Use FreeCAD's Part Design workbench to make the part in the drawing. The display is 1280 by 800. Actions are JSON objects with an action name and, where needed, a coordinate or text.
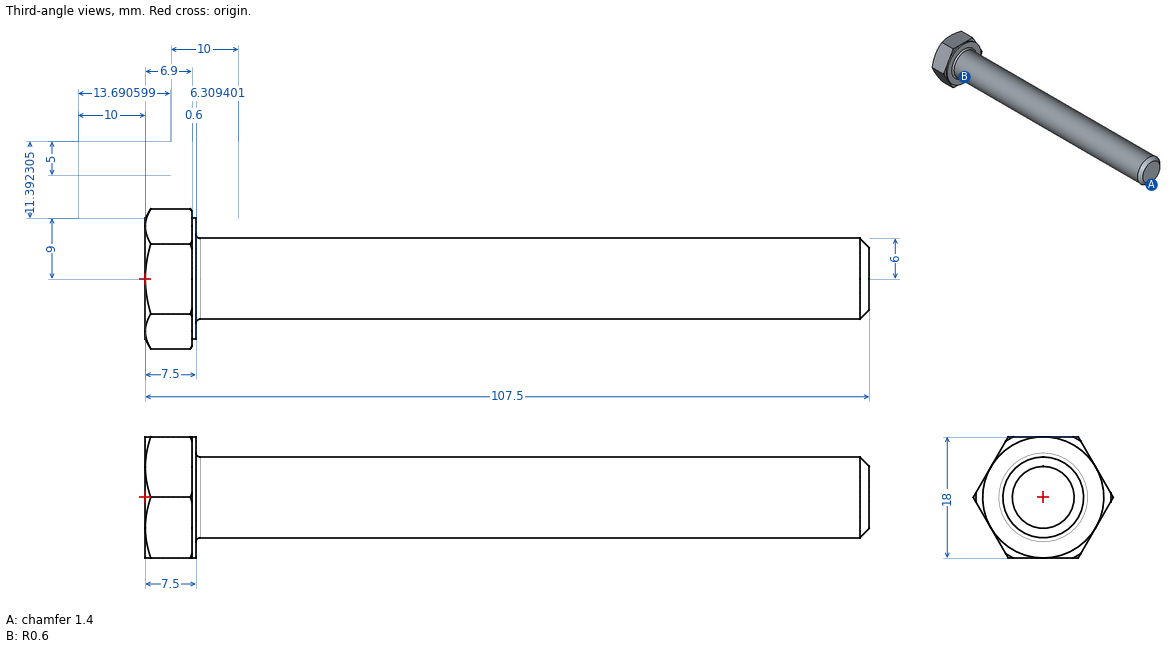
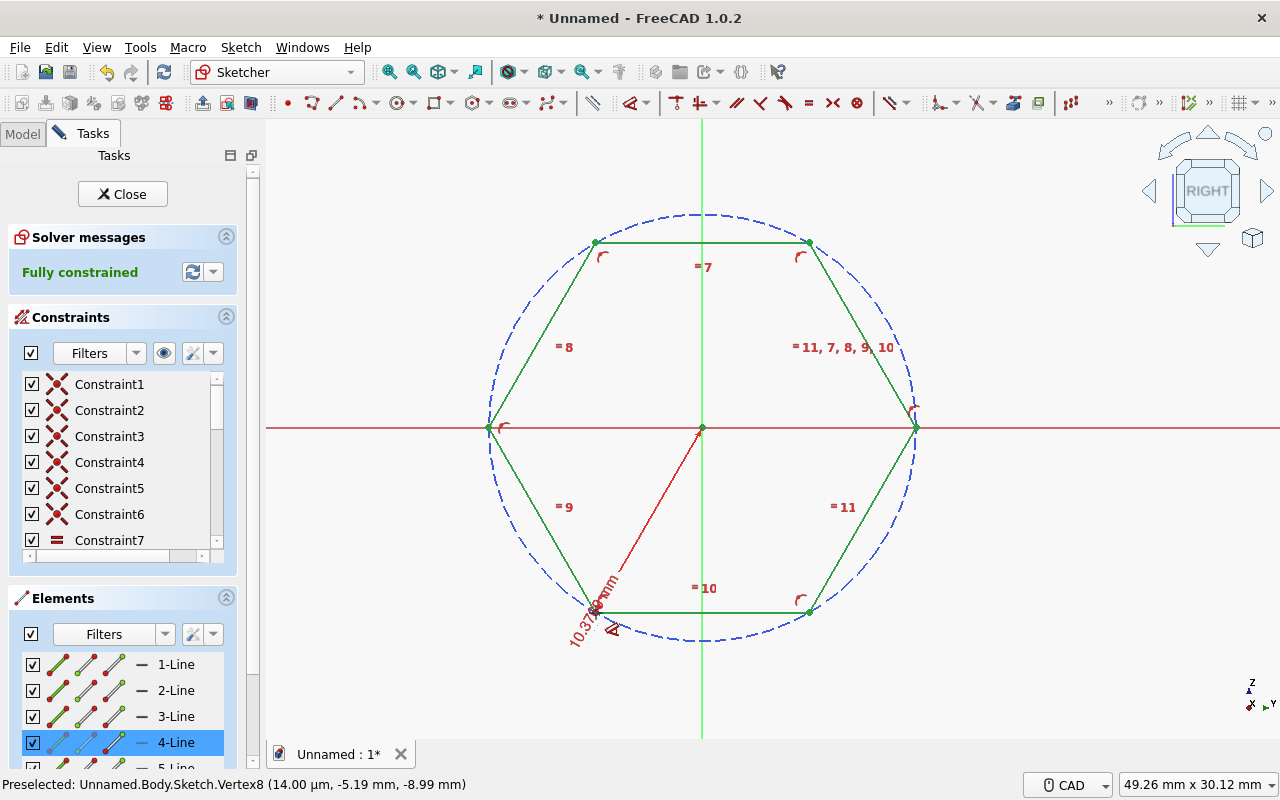
{"action": "left_click", "coordinate": [809, 243]}
{"action": "left_click", "coordinate": [843, 343]}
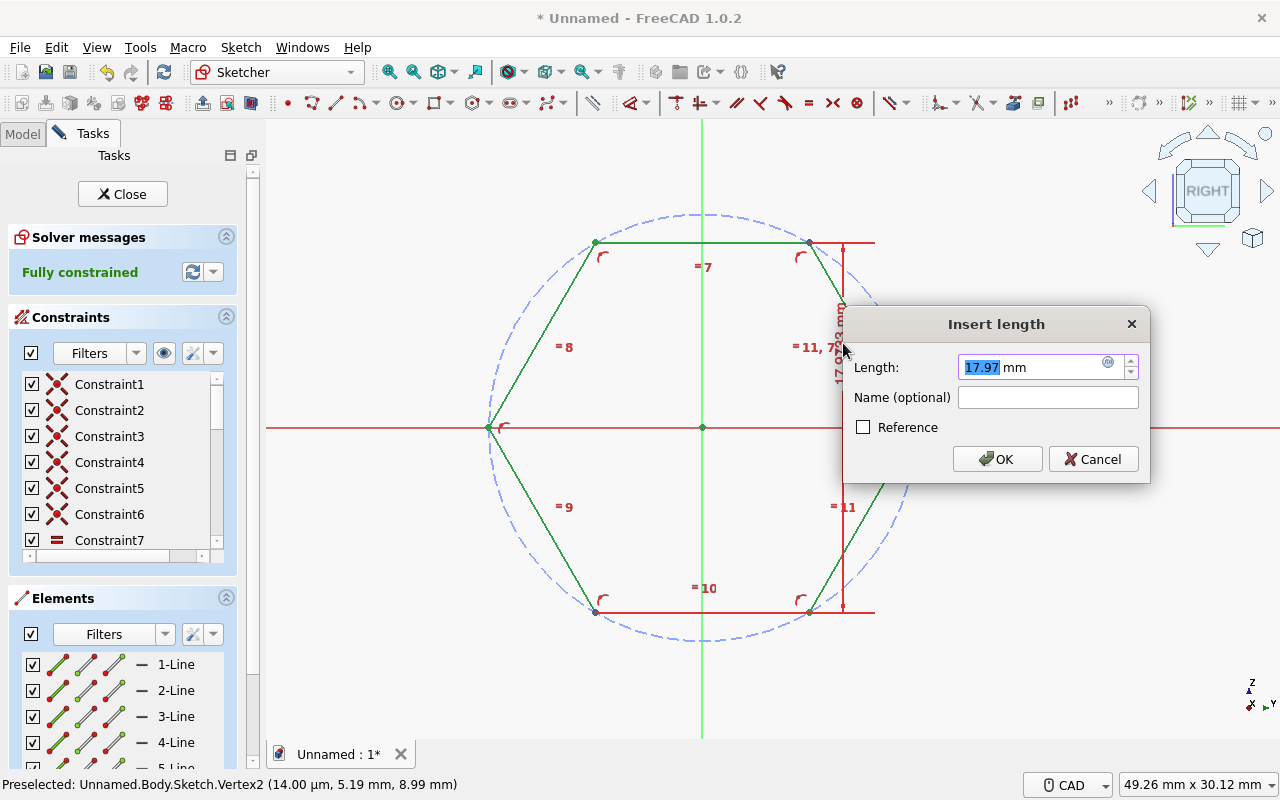
{"action": "type", "text": "18"}
{"action": "key", "text": "Return"}
{"action": "key", "text": "Escape"}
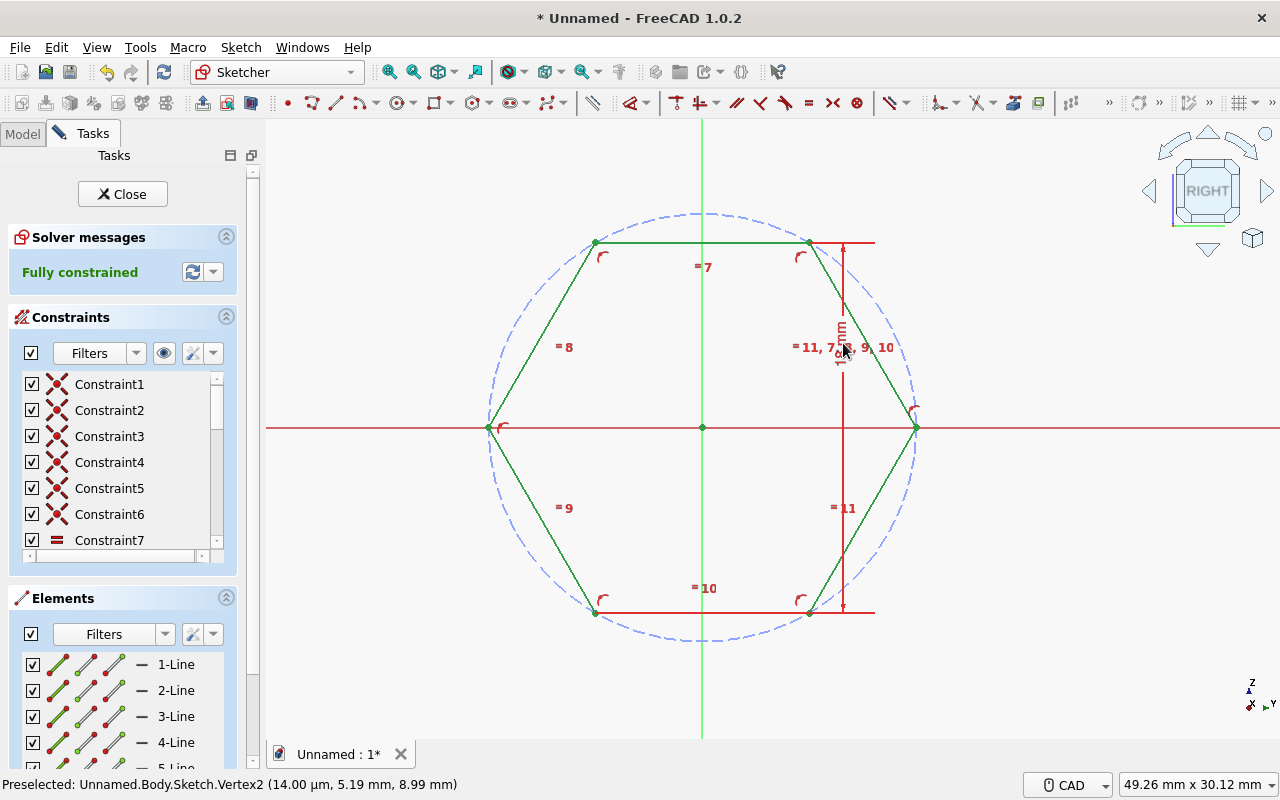
{"action": "left_click", "coordinate": [123, 194]}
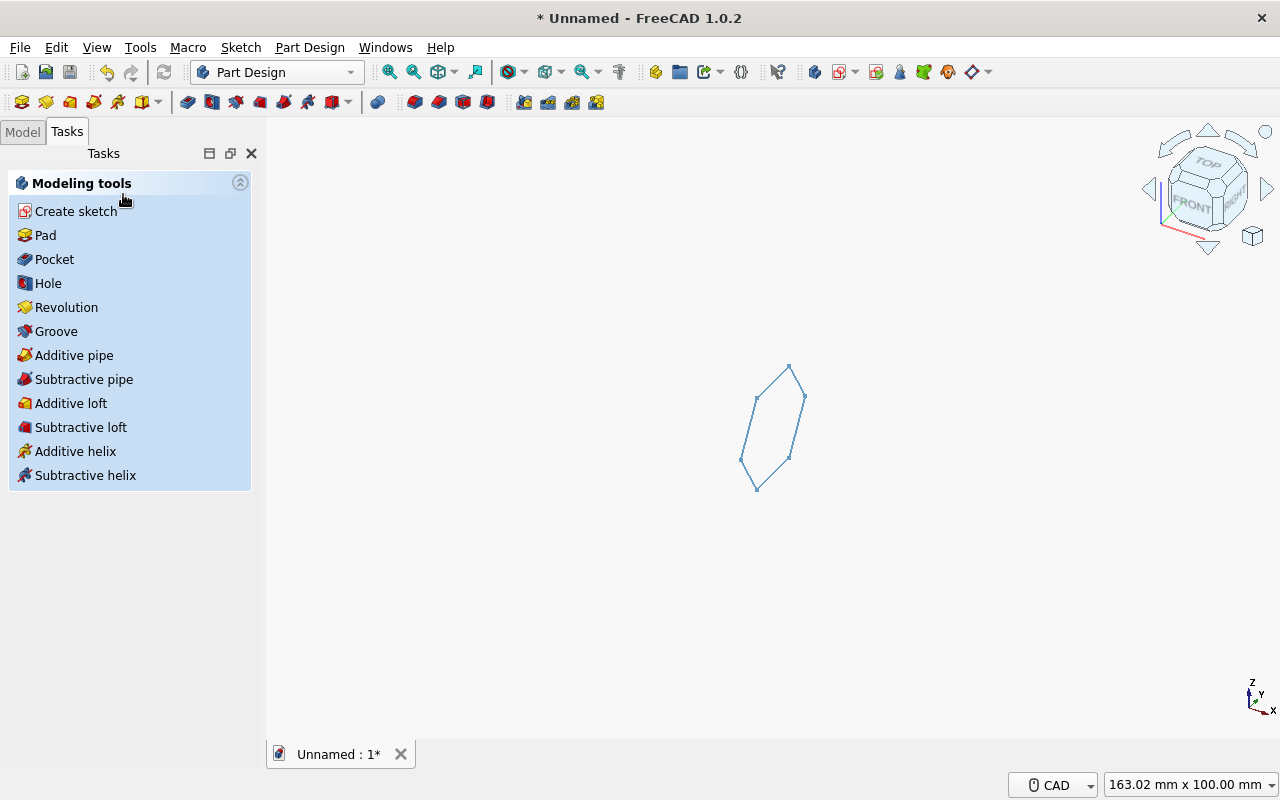
{"action": "left_click", "coordinate": [22, 102]}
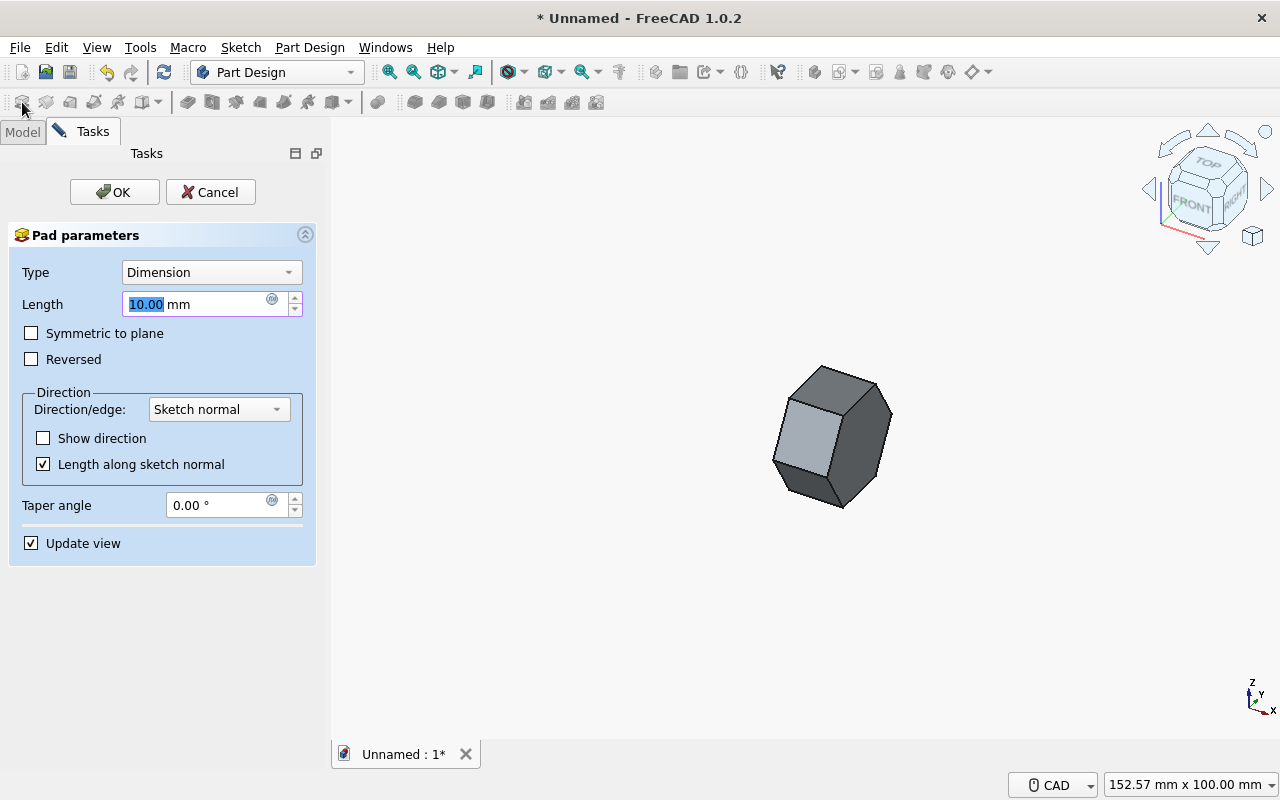
{"action": "type", "text": "7.5"}
{"action": "key", "text": "Tab"}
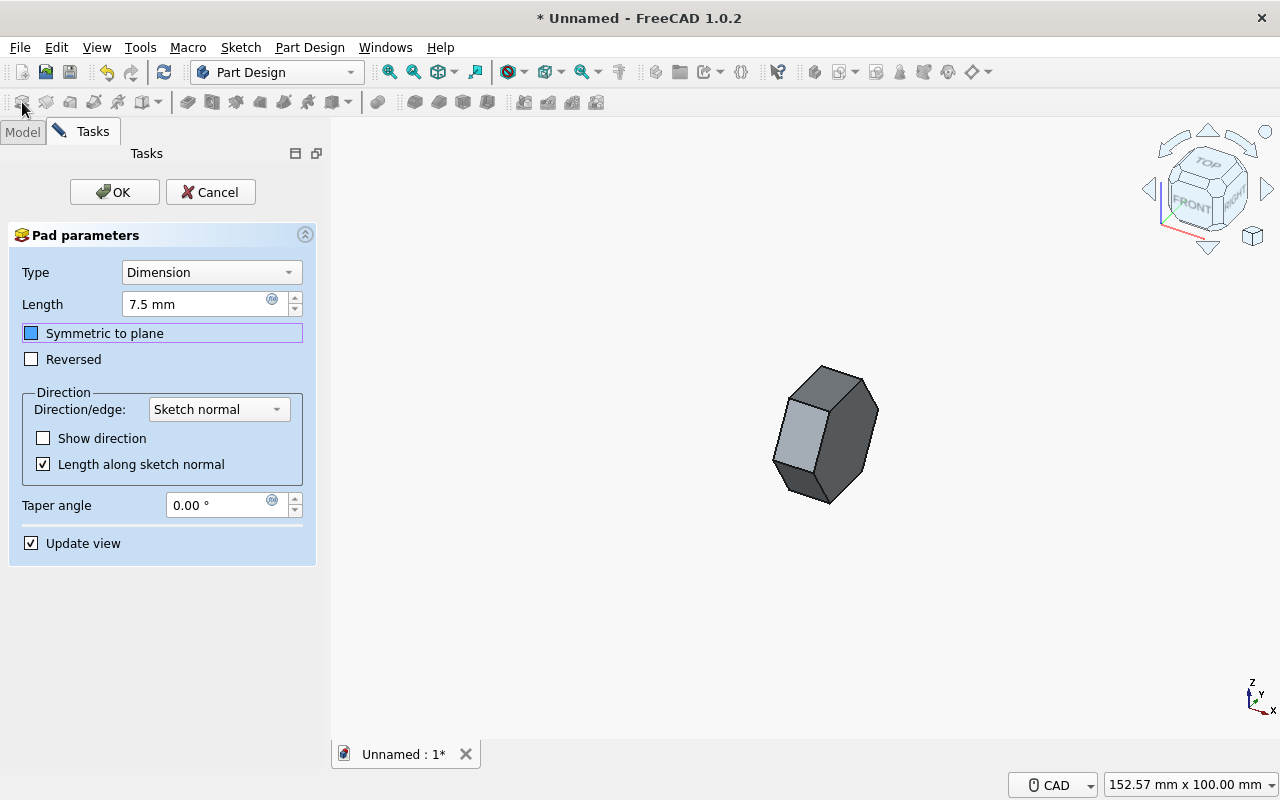
{"action": "left_click", "coordinate": [115, 192]}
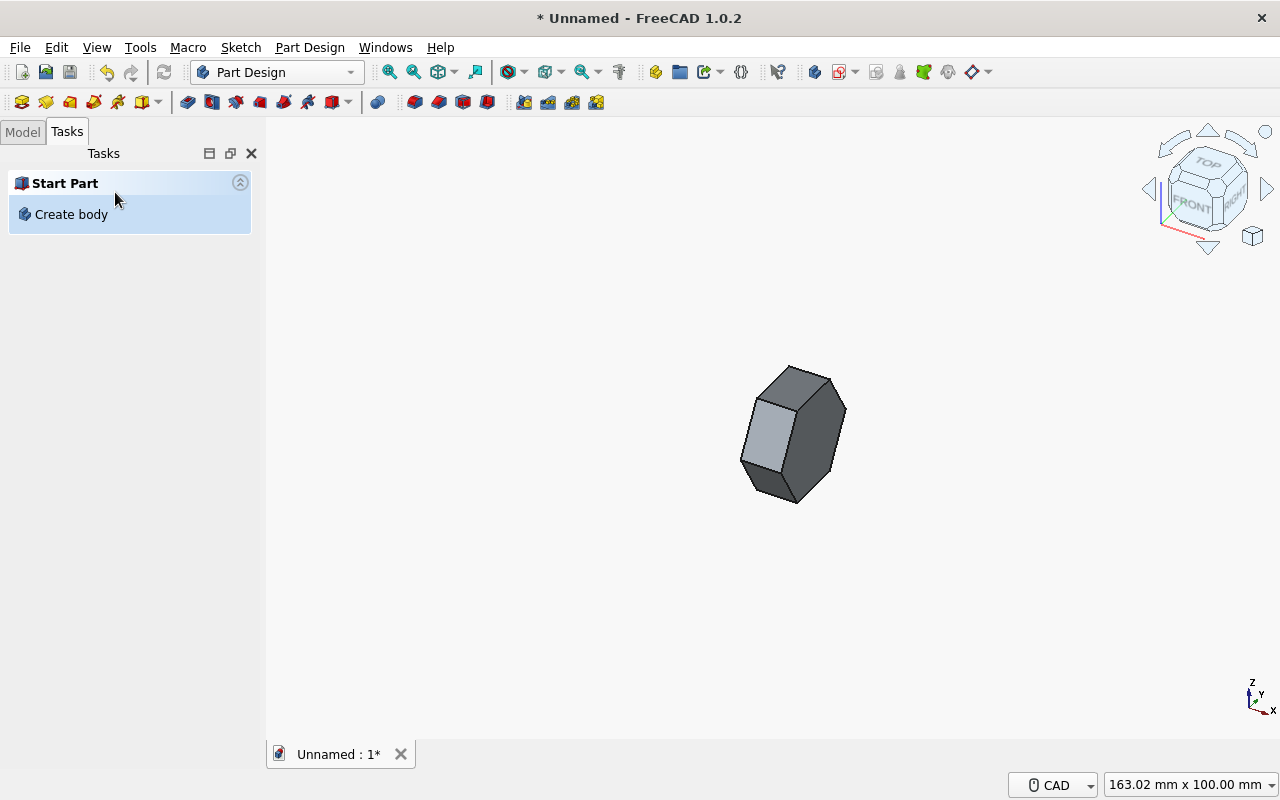
{"action": "key", "text": "v f"}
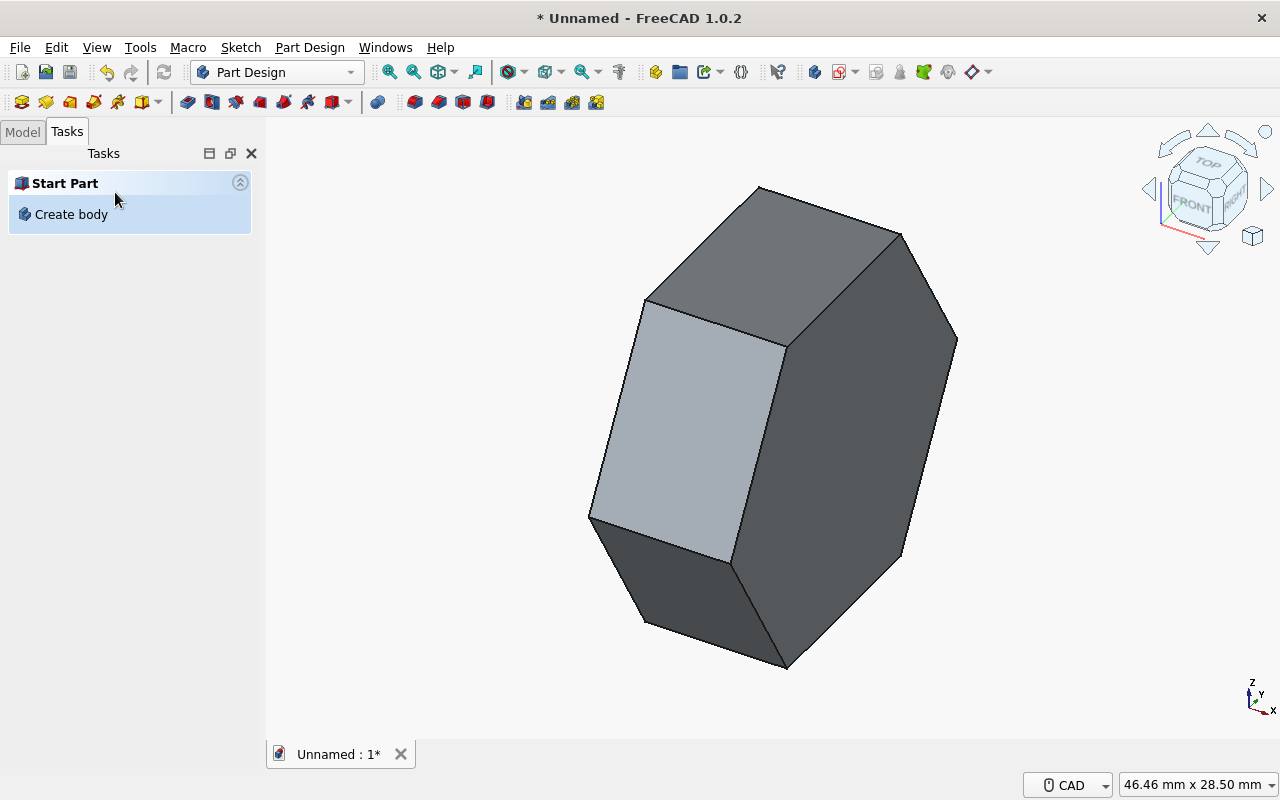
{"action": "left_click", "coordinate": [840, 72]}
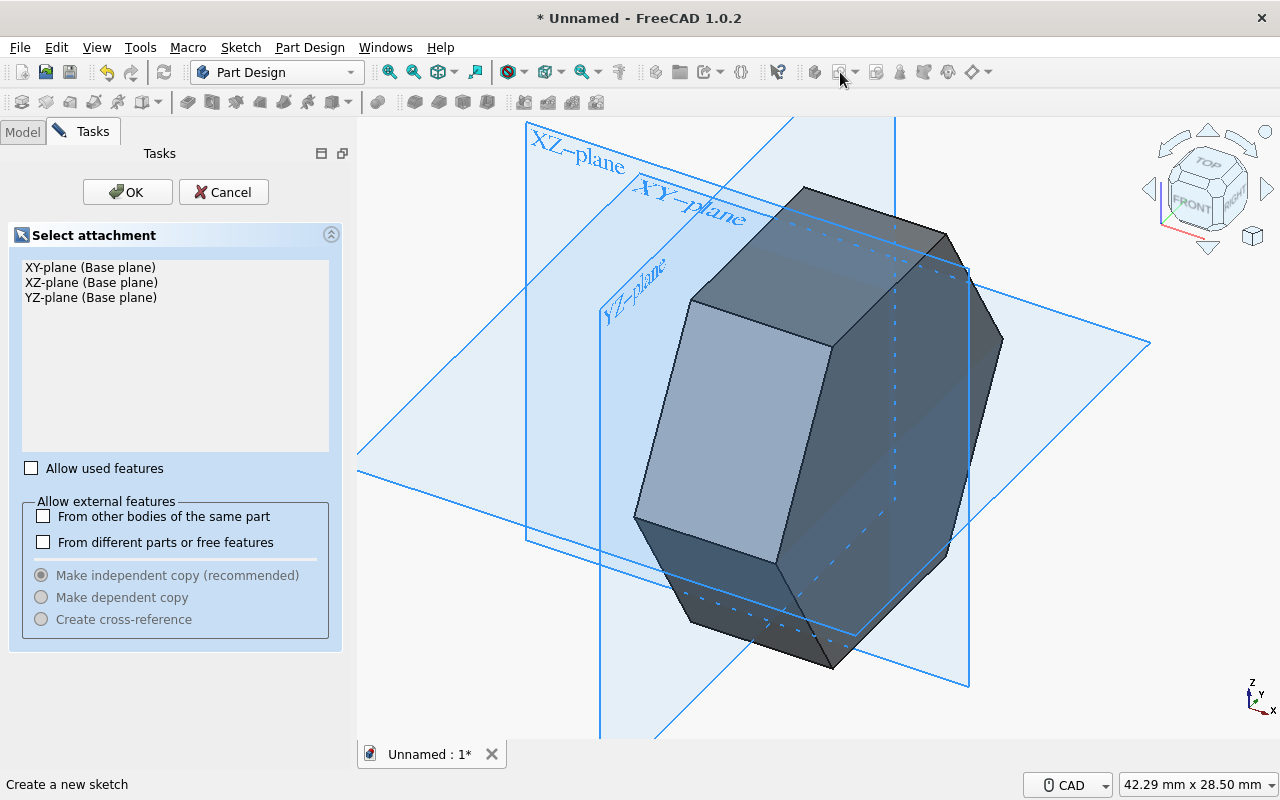
{"action": "left_click", "coordinate": [82, 268]}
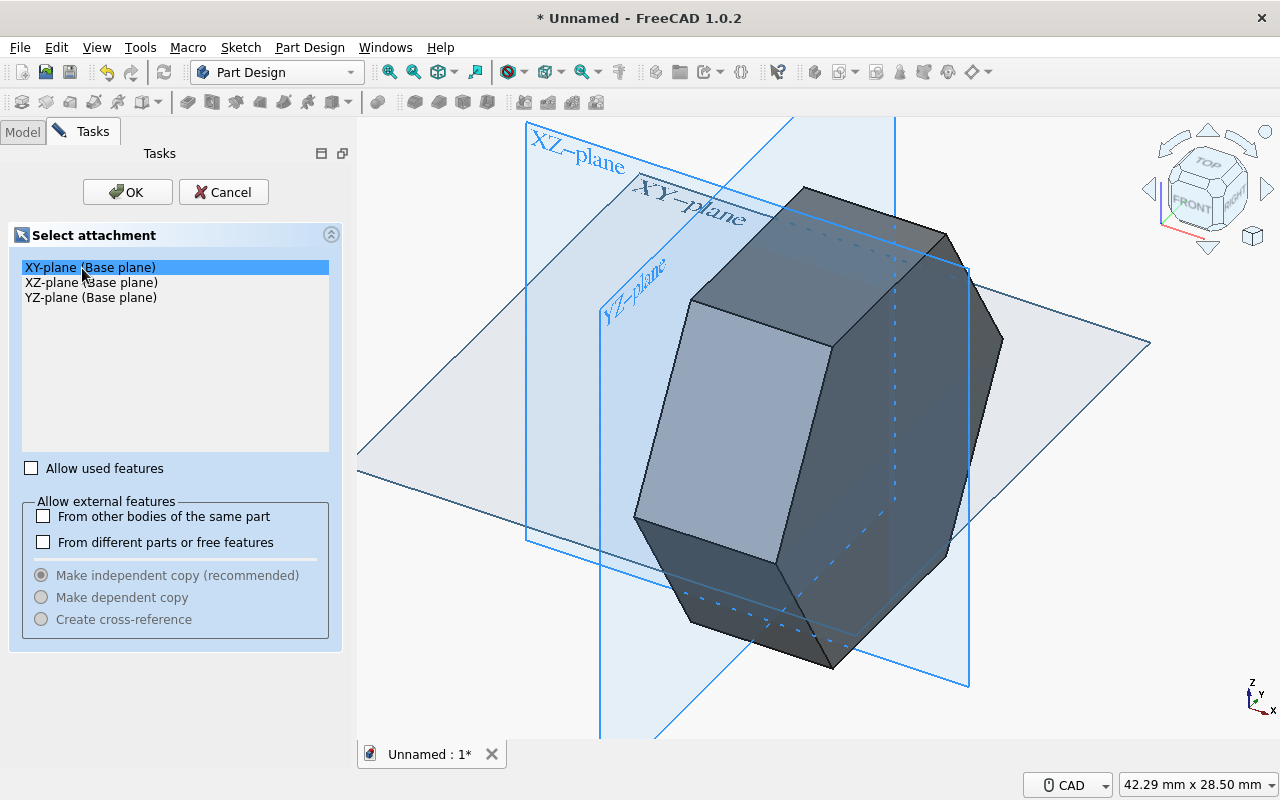
{"action": "left_click", "coordinate": [128, 192]}